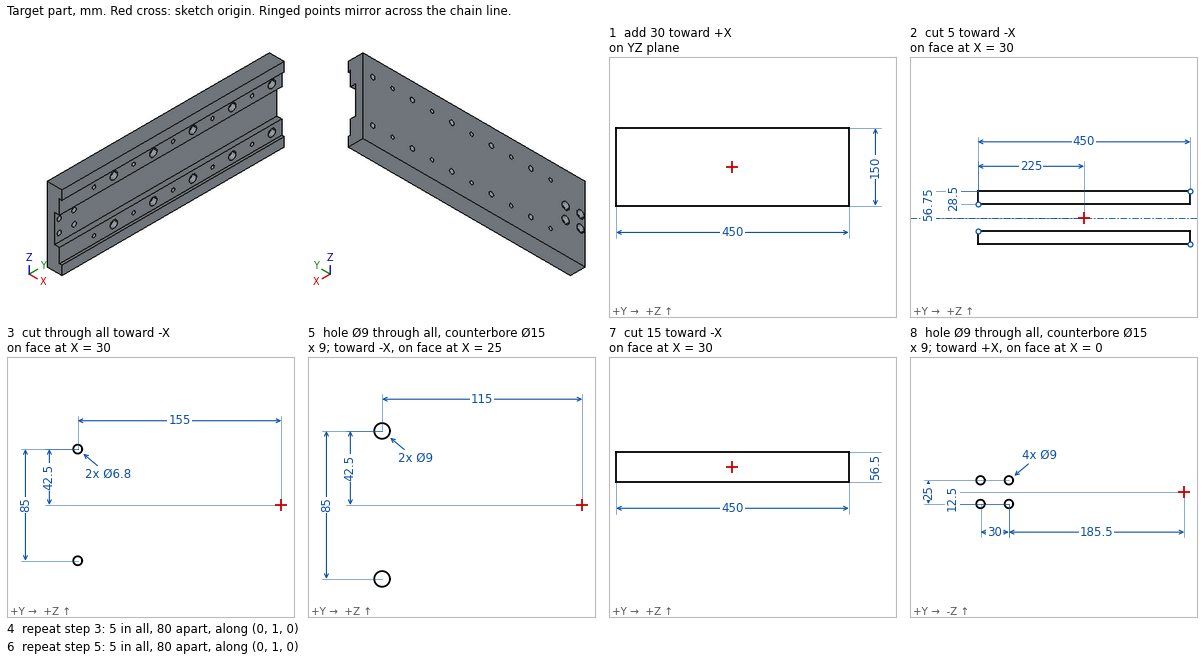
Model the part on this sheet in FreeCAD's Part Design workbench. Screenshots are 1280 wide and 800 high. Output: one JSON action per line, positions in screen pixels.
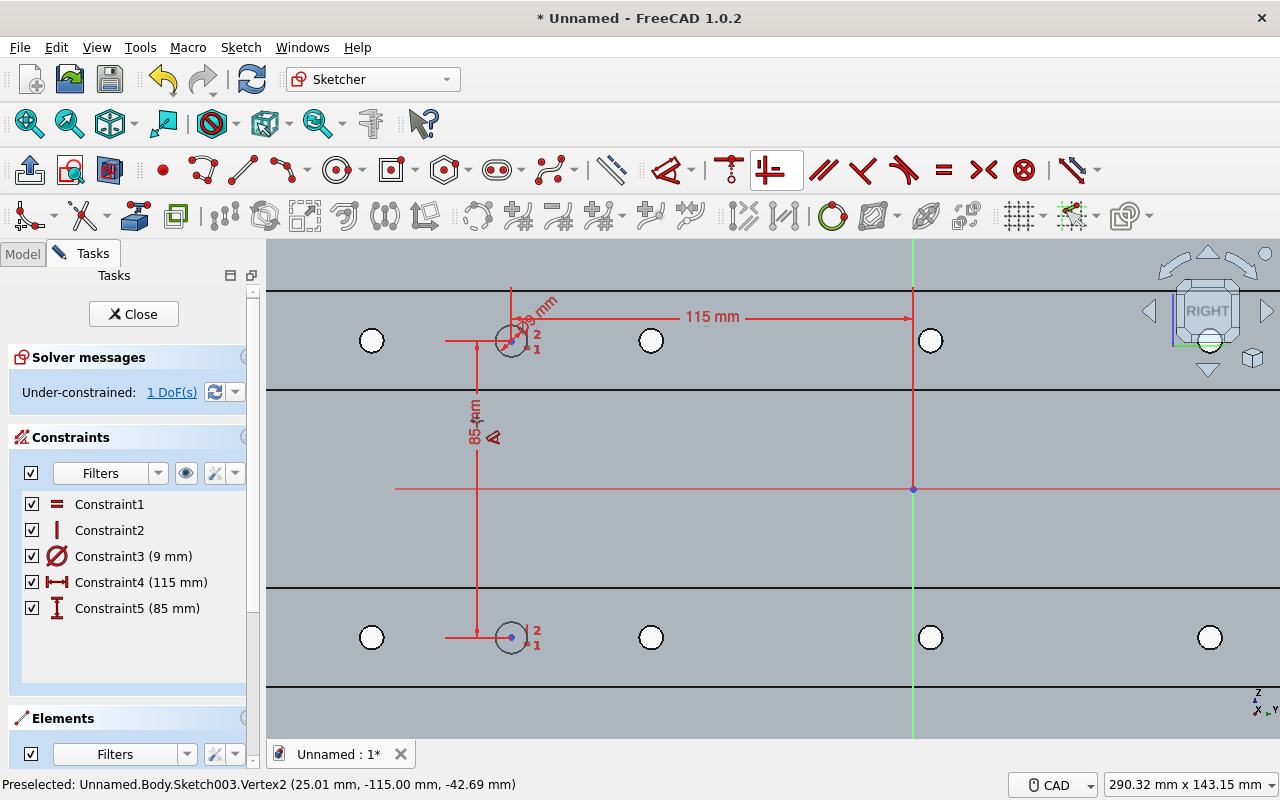
{"action": "left_click", "coordinate": [511, 341]}
{"action": "left_click", "coordinate": [947, 415]}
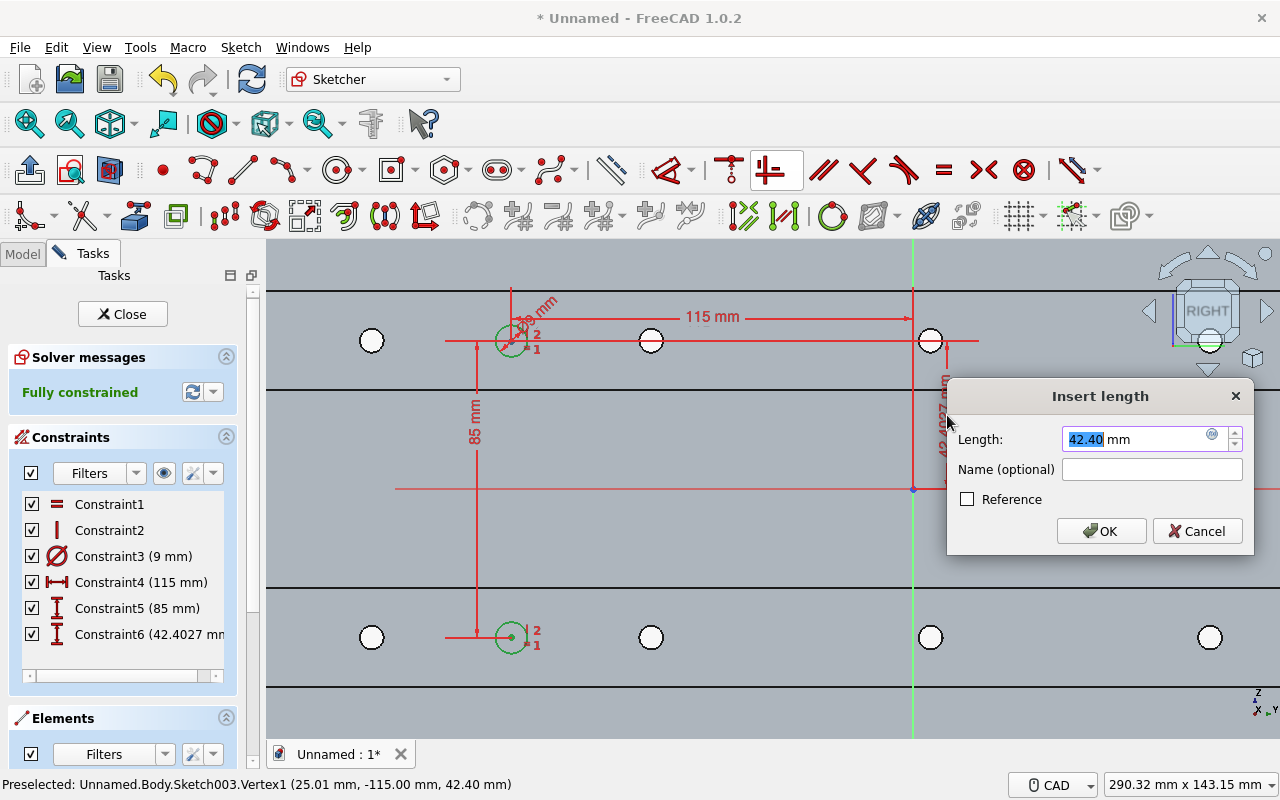
{"action": "type", "text": "42.5"}
{"action": "key", "text": "Return"}
{"action": "key", "text": "Escape"}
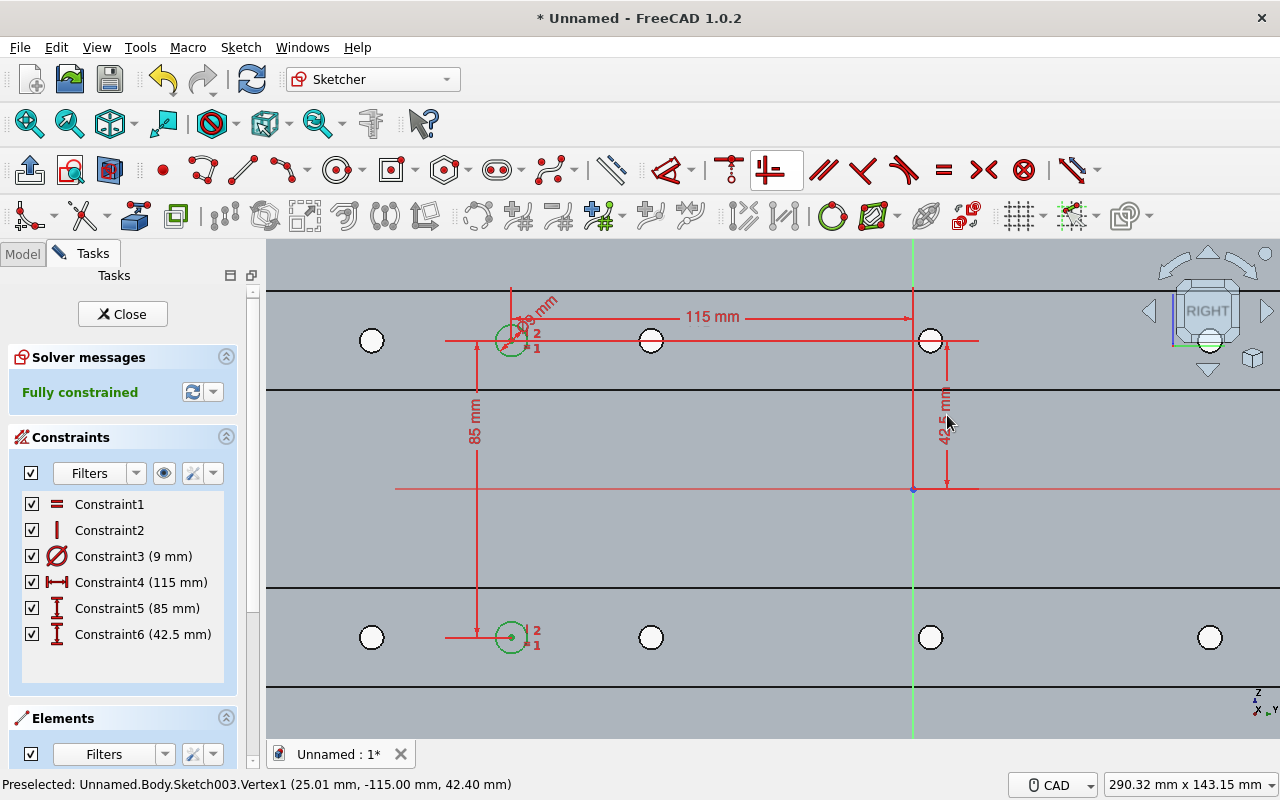
{"action": "left_click", "coordinate": [123, 314]}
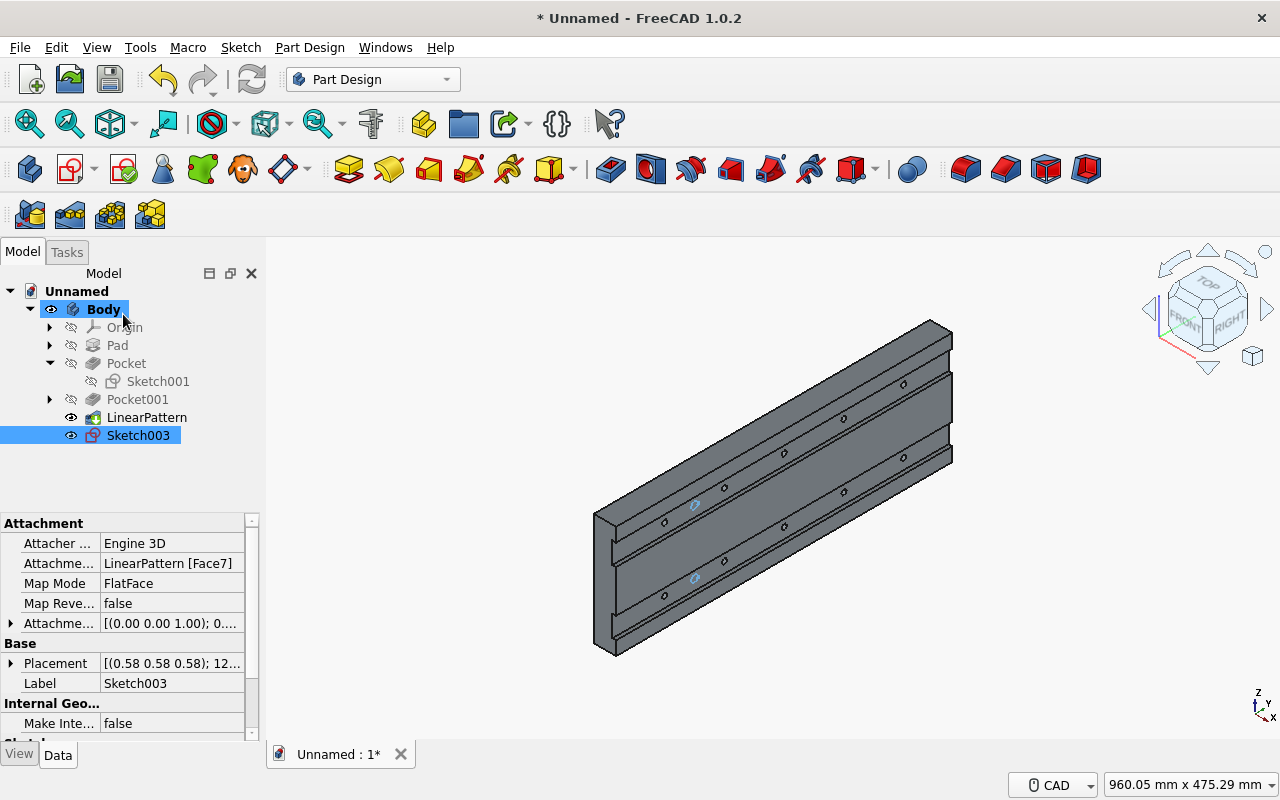
{"action": "left_click", "coordinate": [652, 170]}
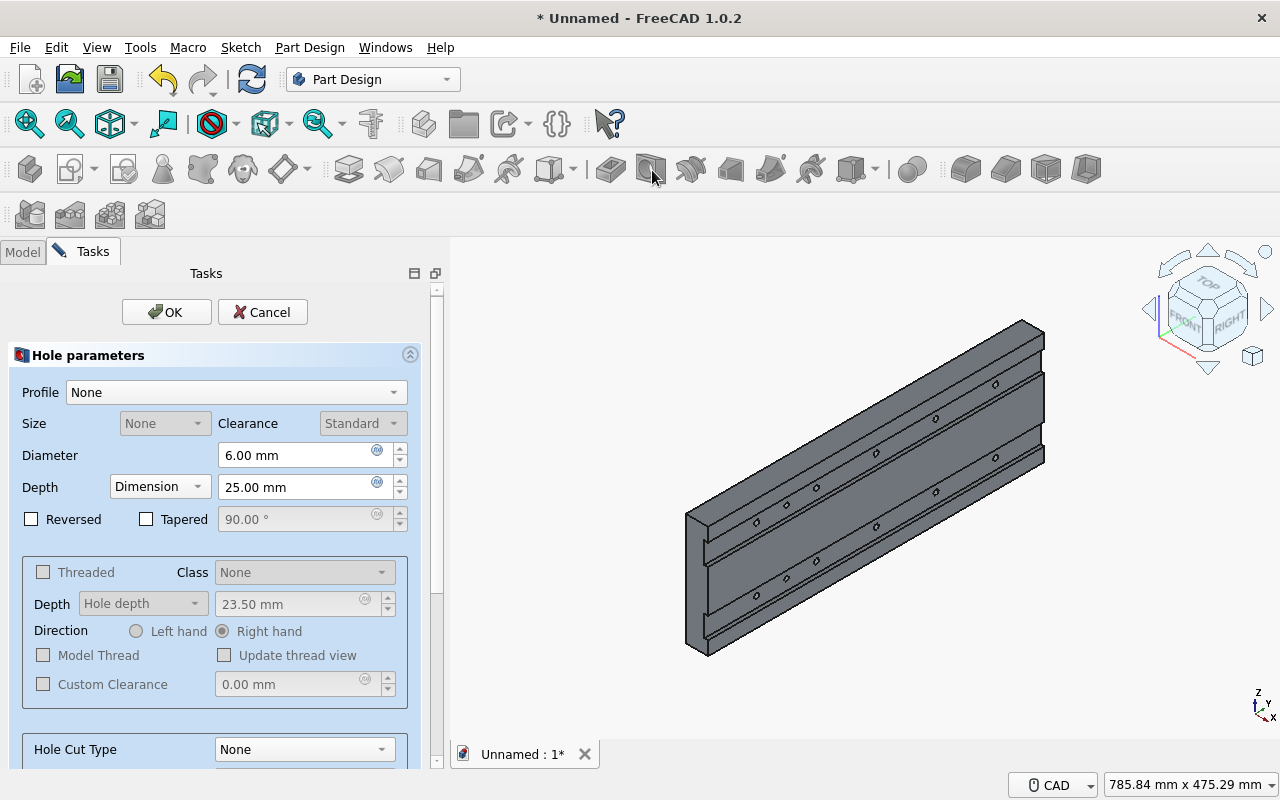
{"action": "triple_click", "coordinate": [305, 455]}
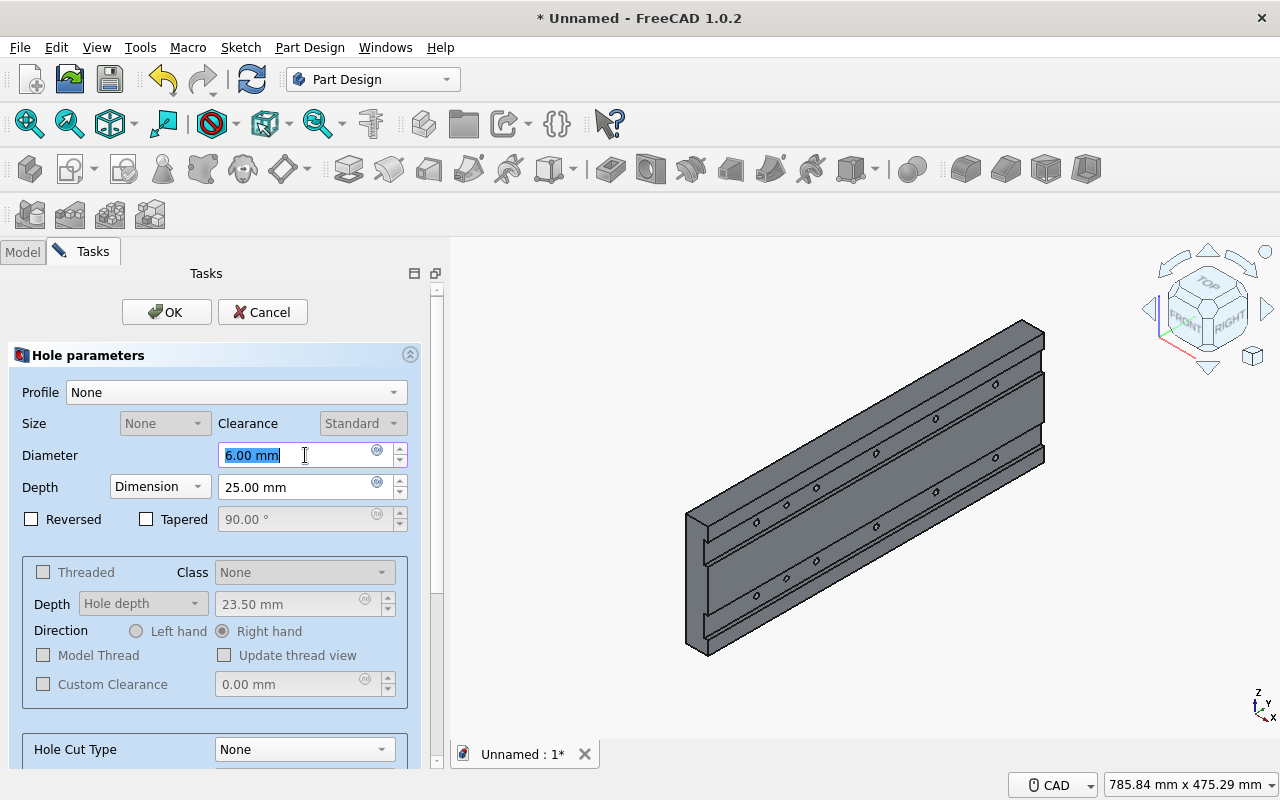
{"action": "type", "text": "9"}
{"action": "key", "text": "Tab"}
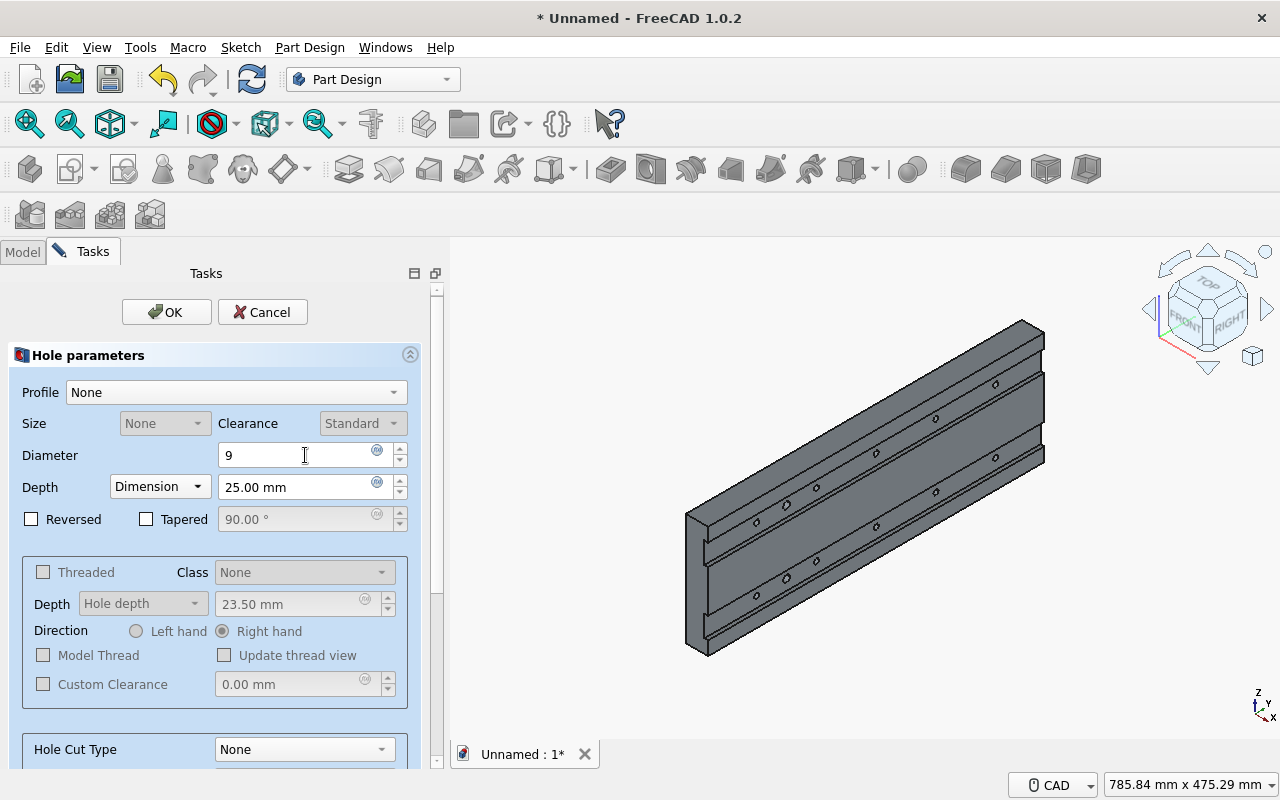
{"action": "left_click", "coordinate": [161, 486]}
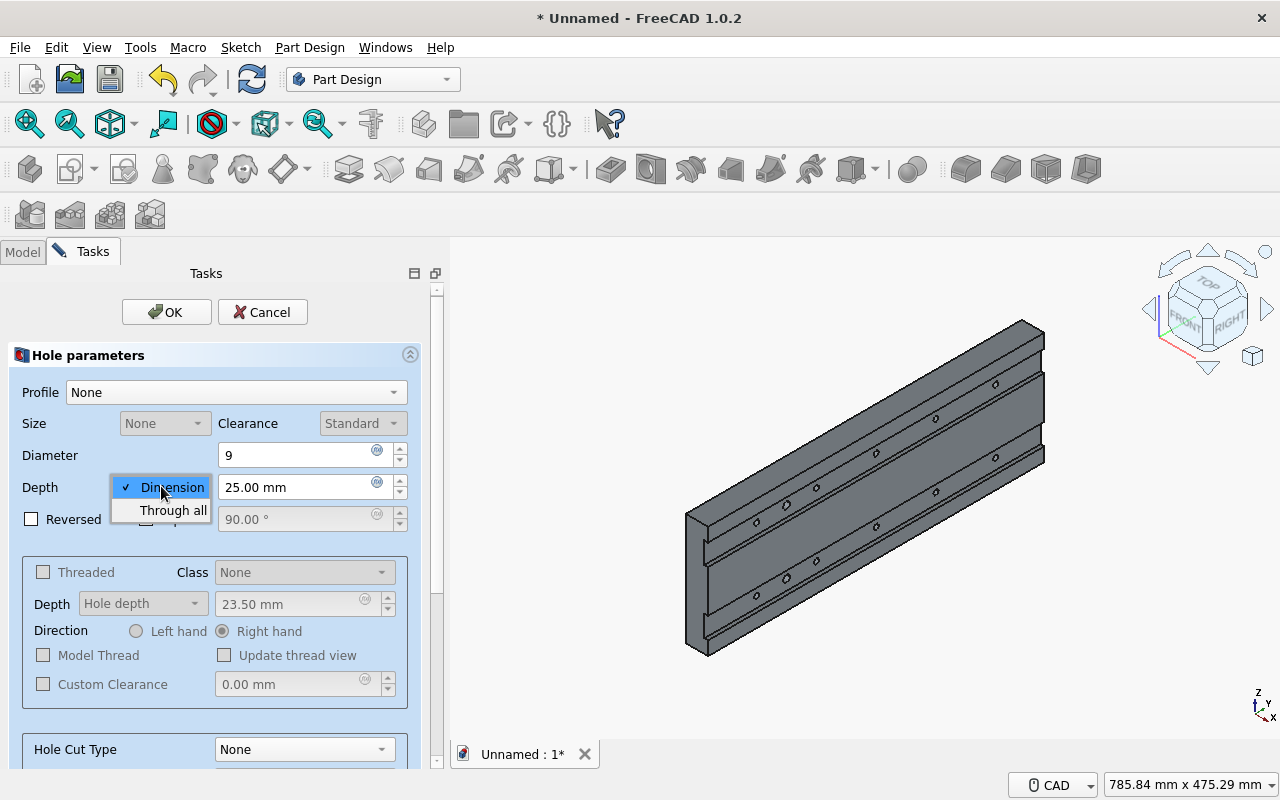
{"action": "left_click", "coordinate": [160, 510]}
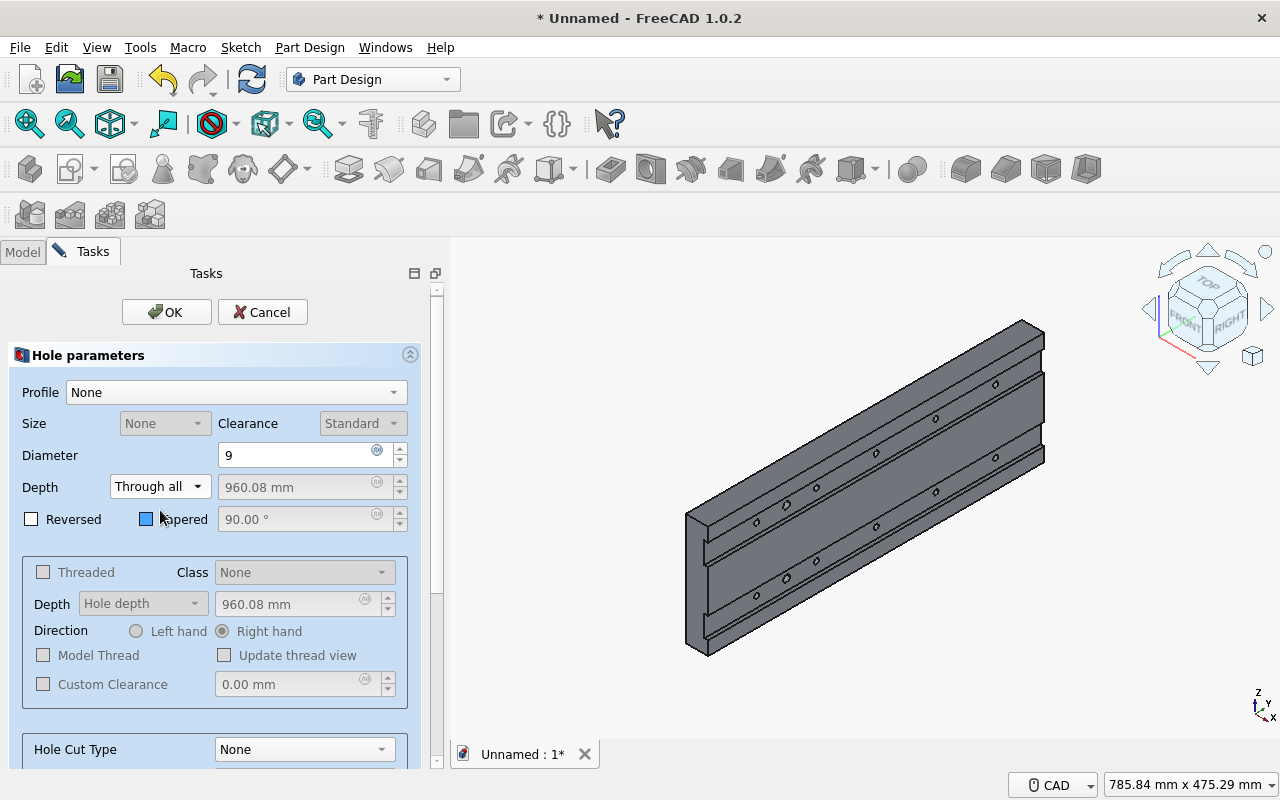
{"action": "left_click", "coordinate": [306, 750]}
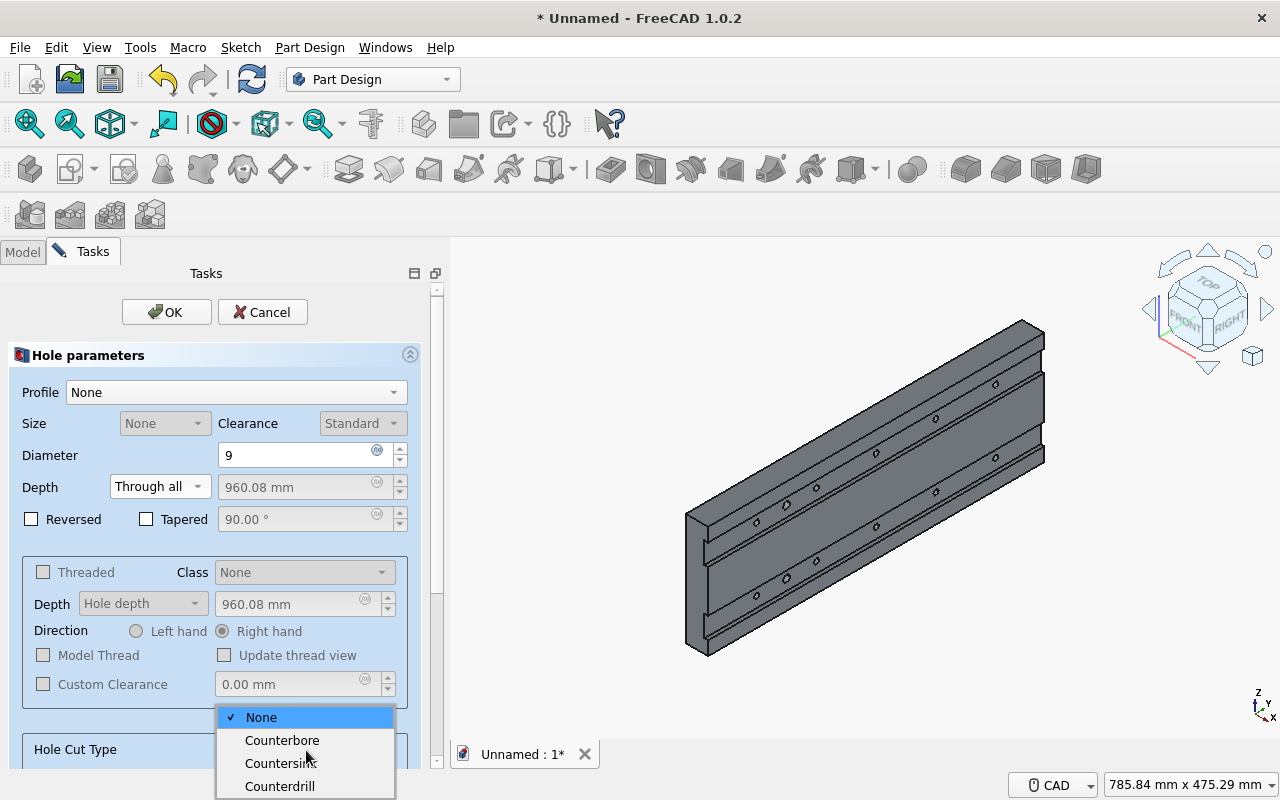
{"action": "left_click", "coordinate": [304, 740]}